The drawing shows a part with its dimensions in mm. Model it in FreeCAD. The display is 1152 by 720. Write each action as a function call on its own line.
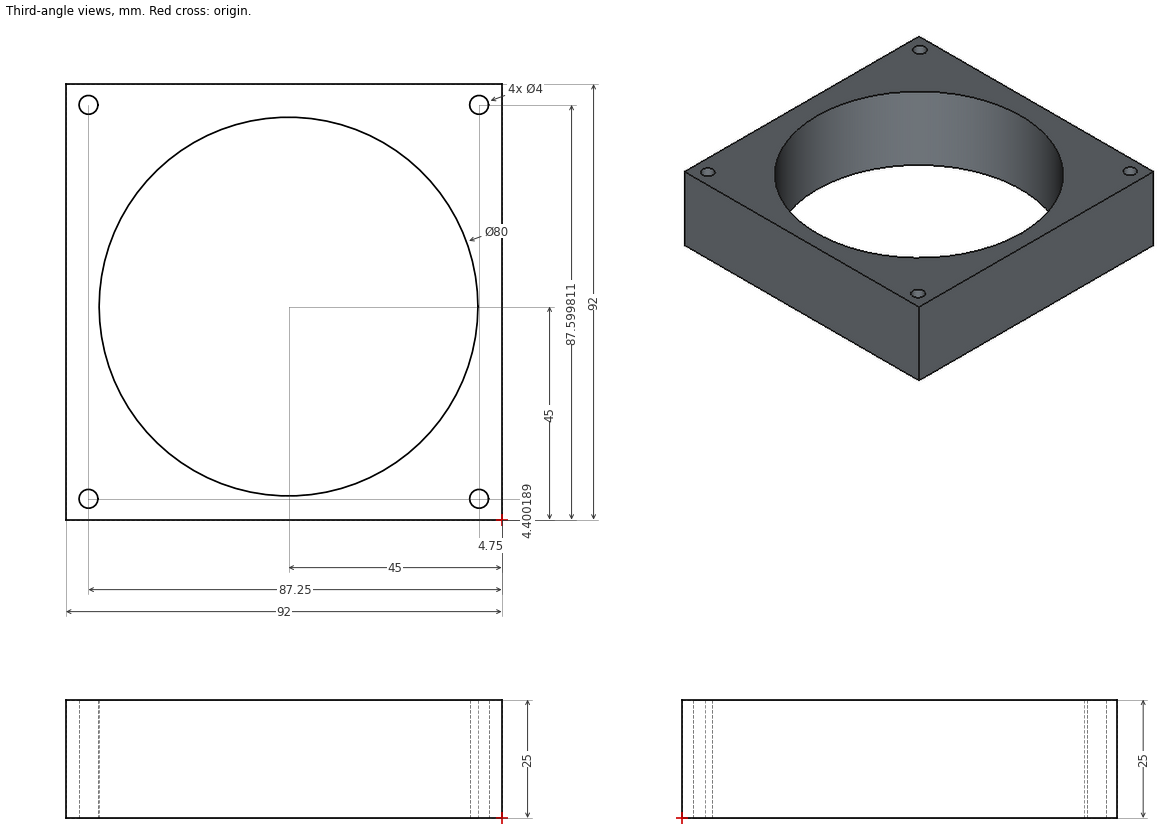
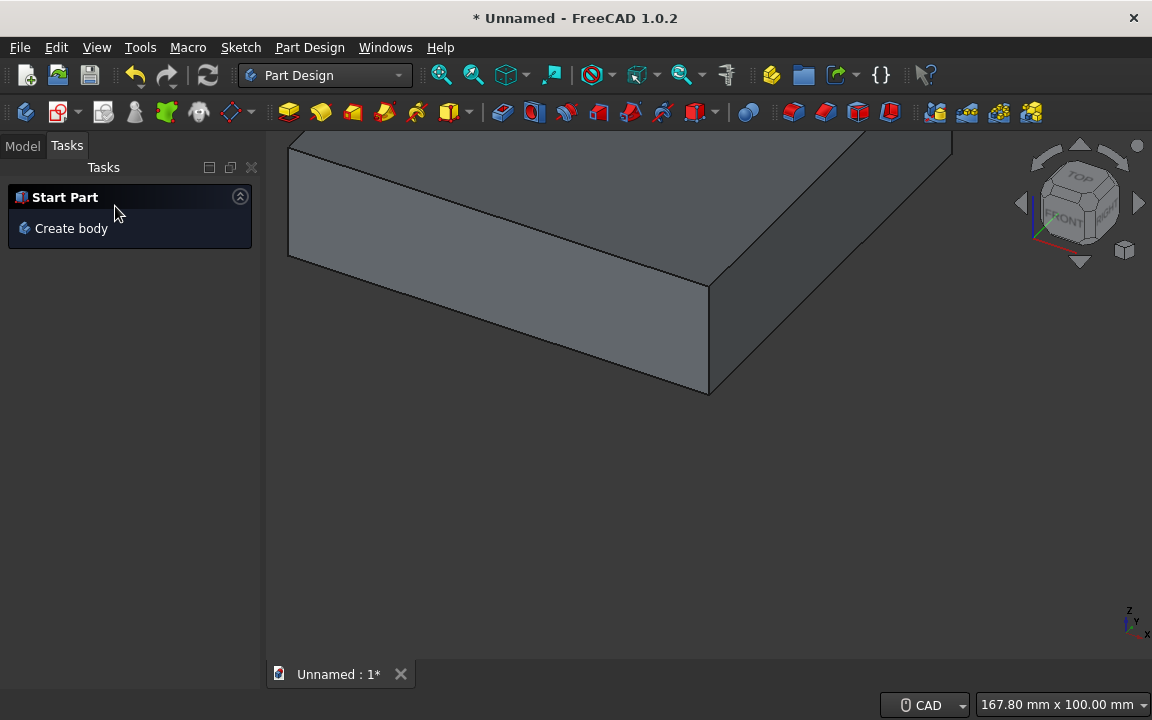
key(v)
key(f)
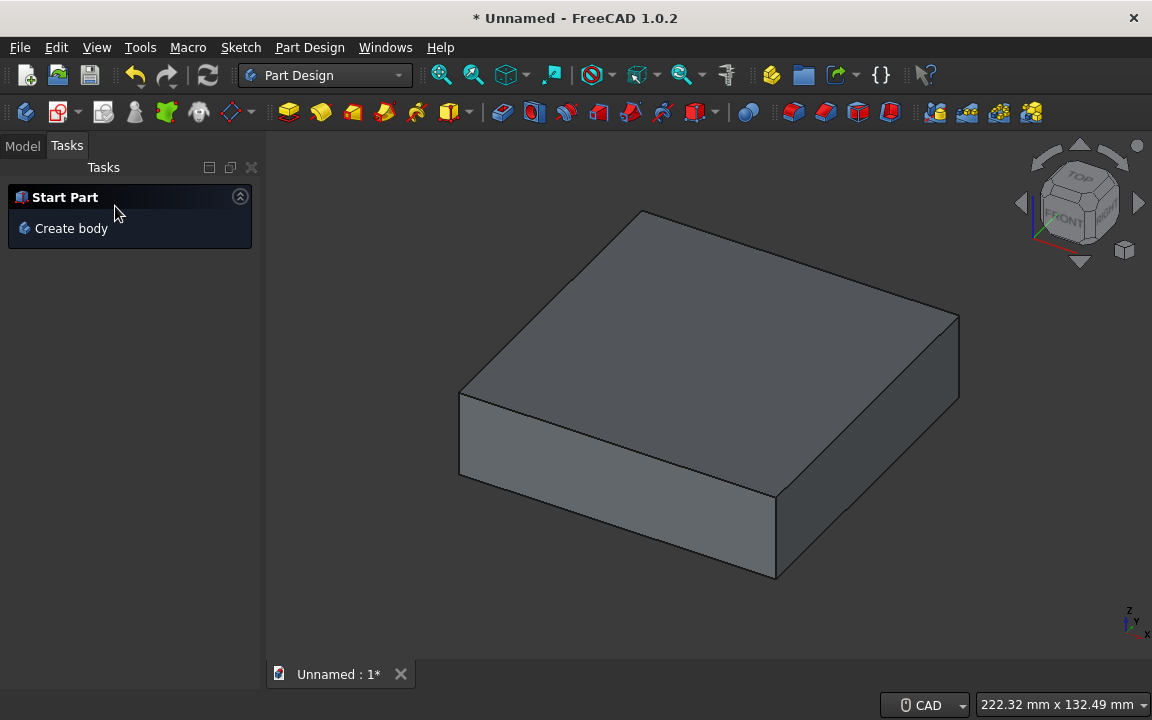
click(709, 353)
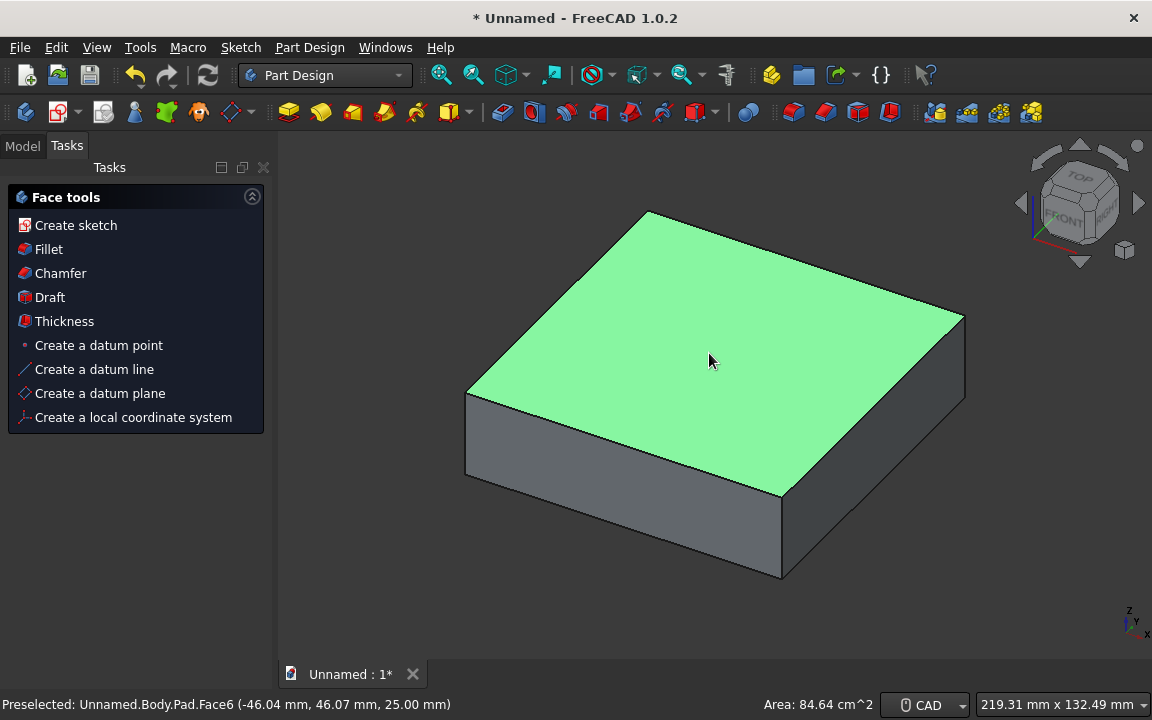
click(58, 112)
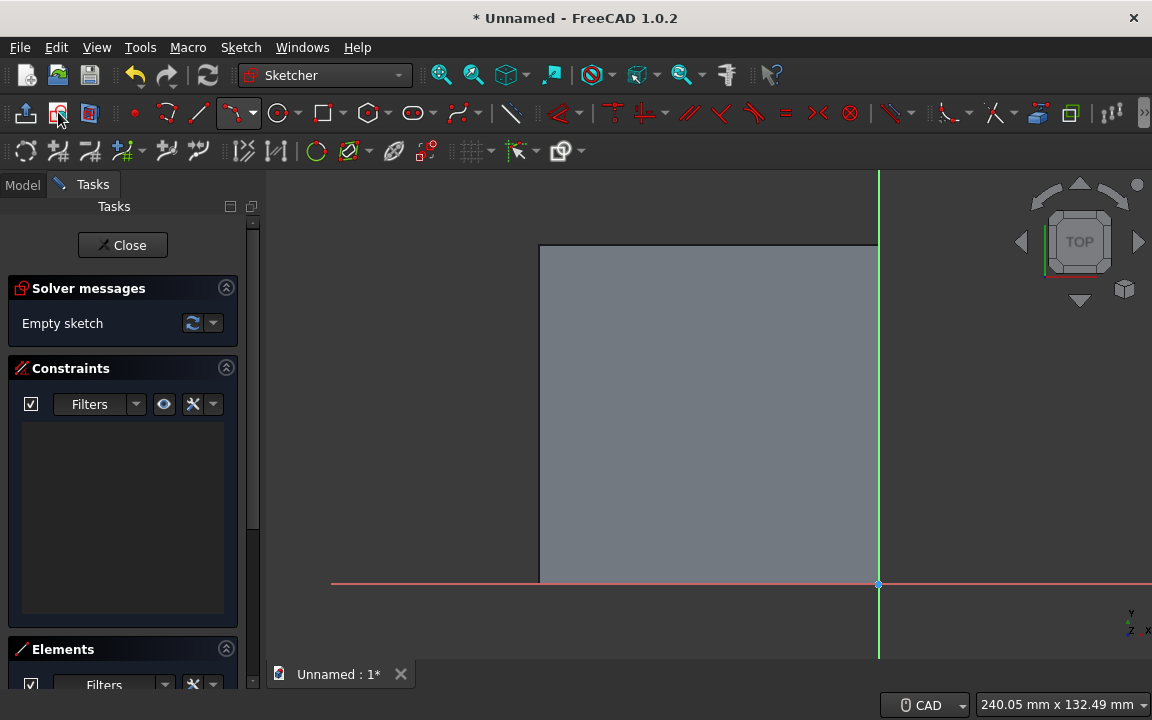
click(278, 114)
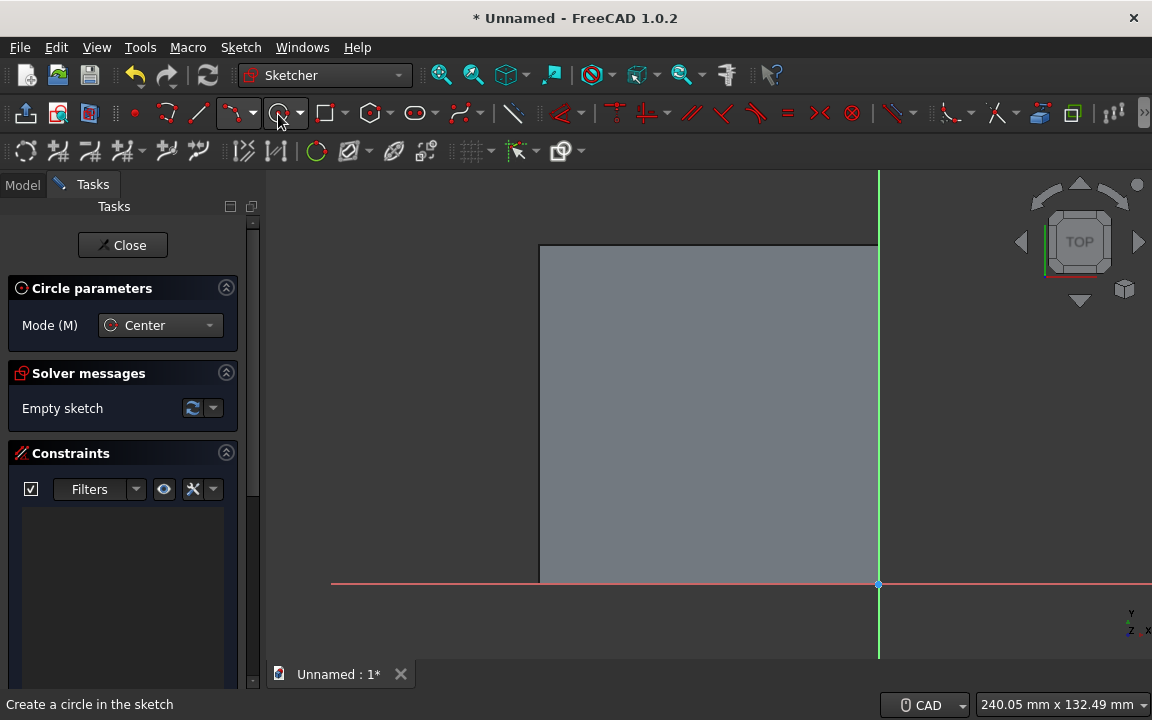
click(713, 418)
move(817, 314)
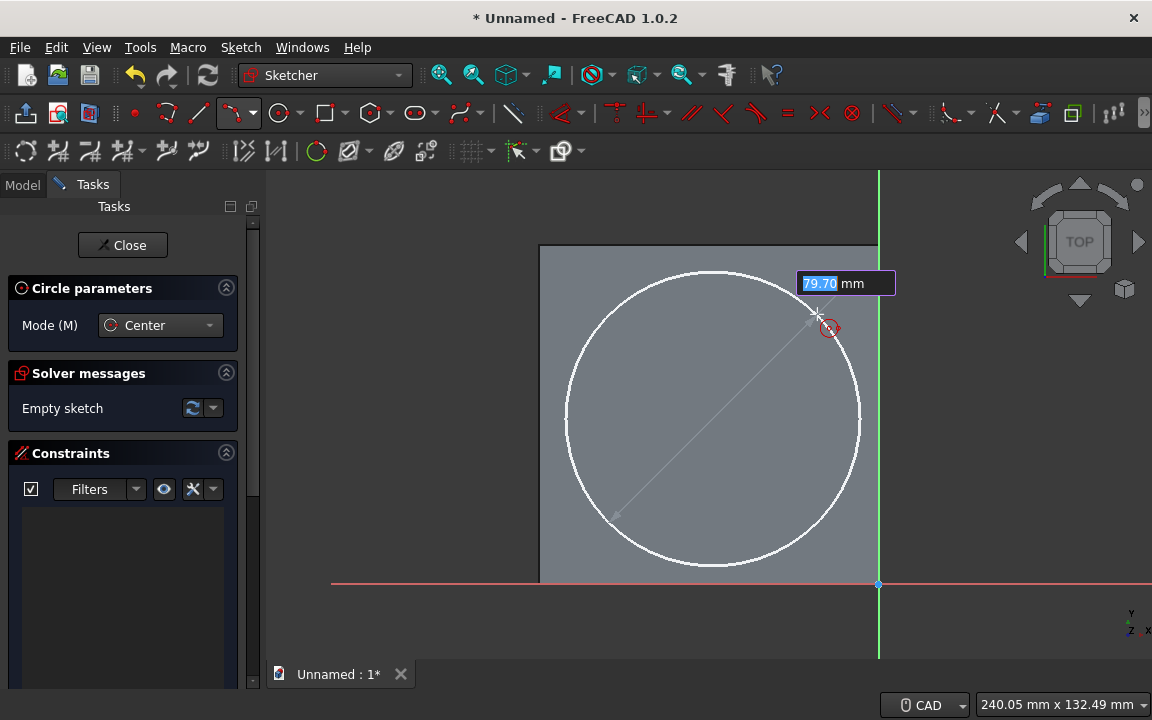
text(80)
key(Return)
key(Escape)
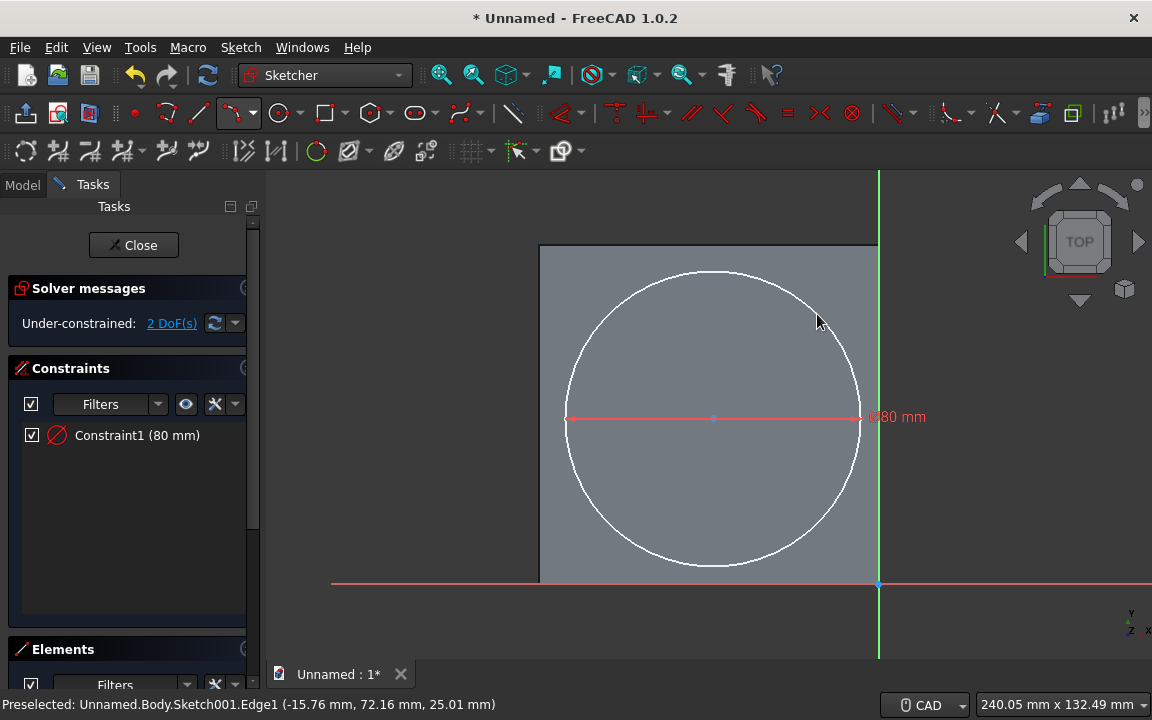
click(713, 419)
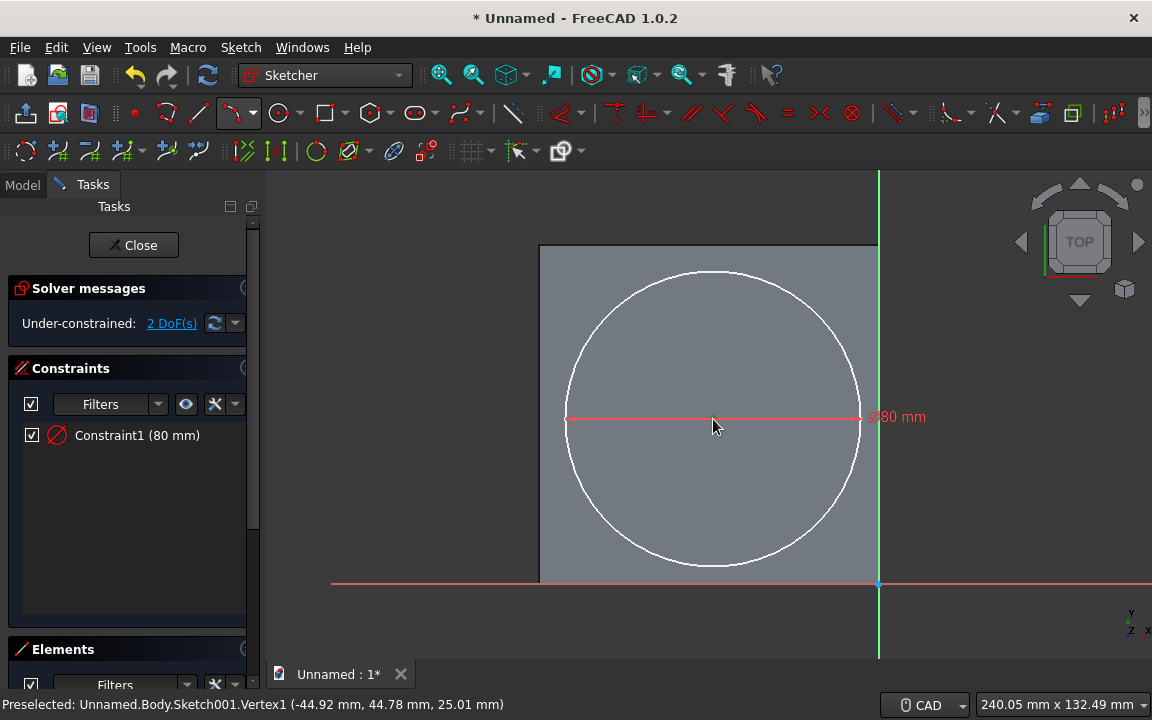
click(584, 114)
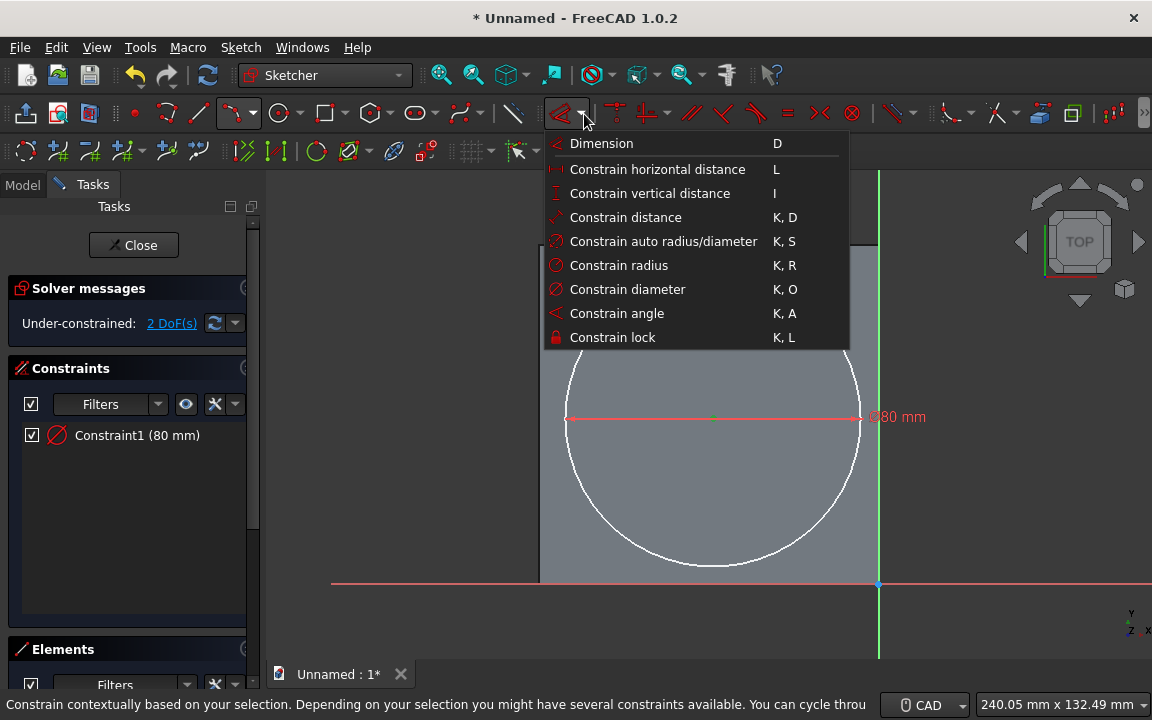
click(697, 169)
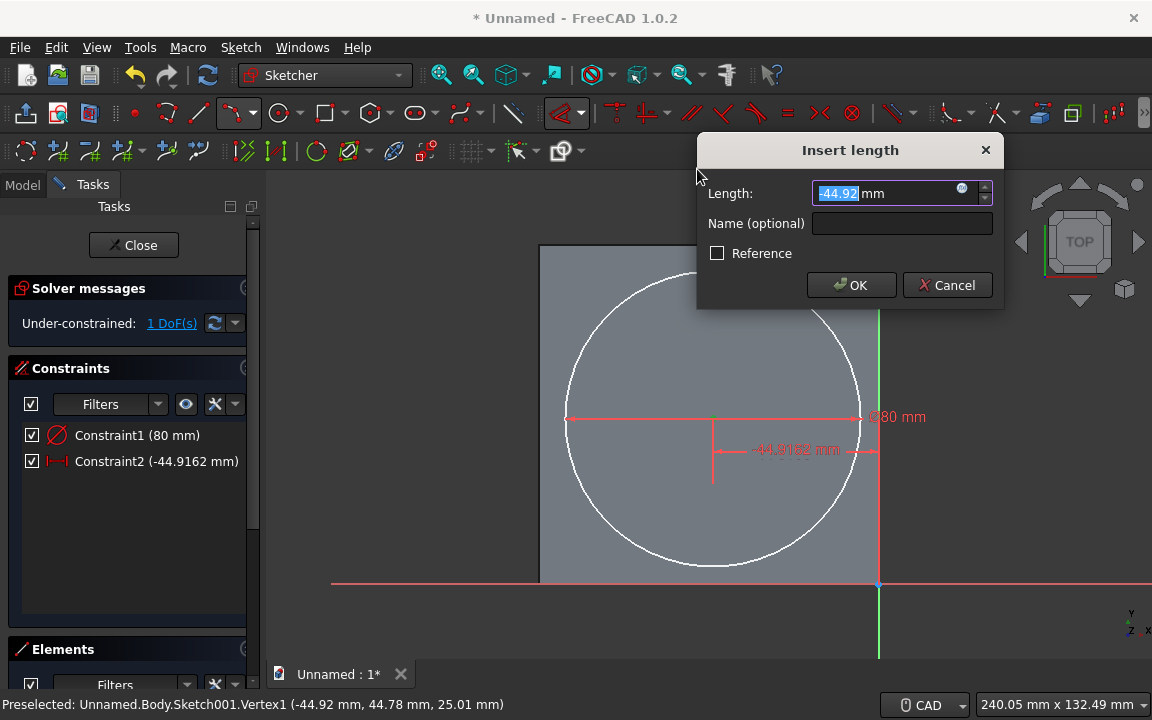
text(-45)
key(Return)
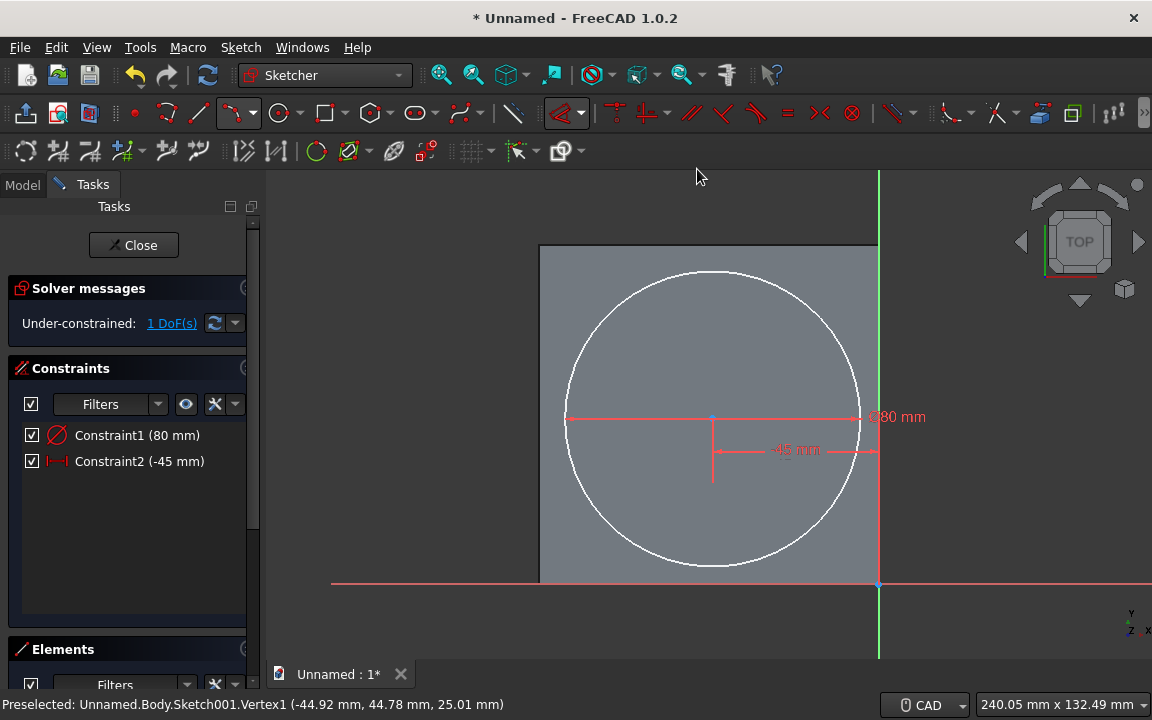
click(713, 419)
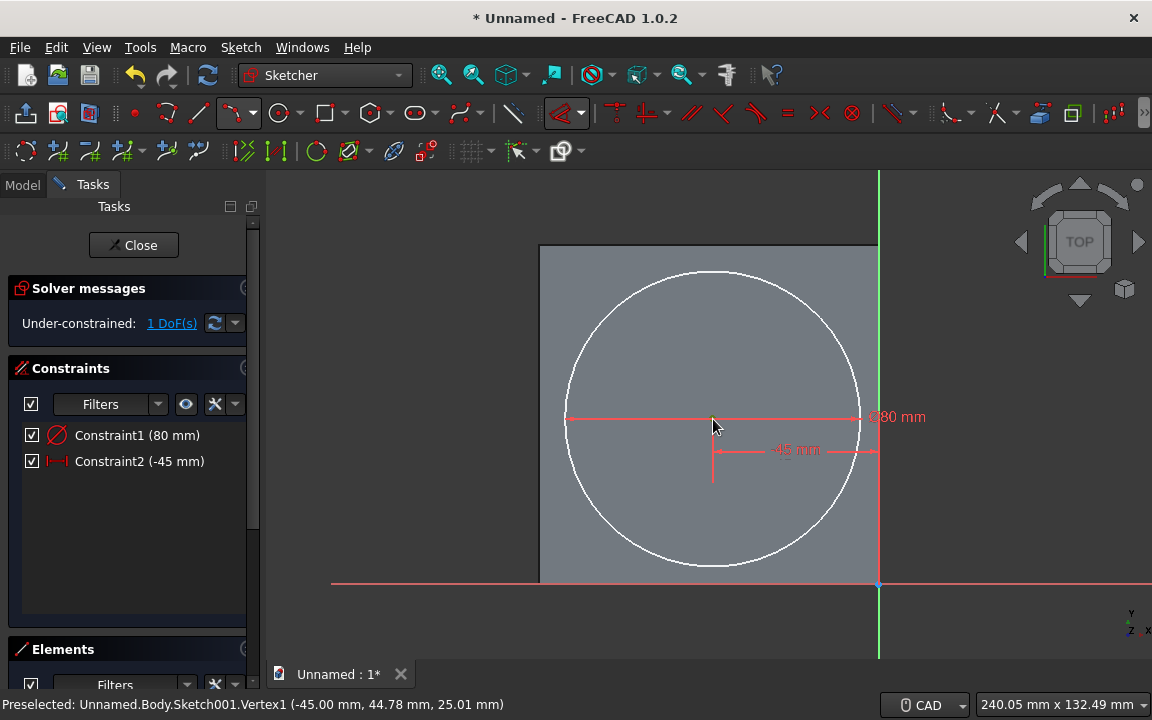
key(i)